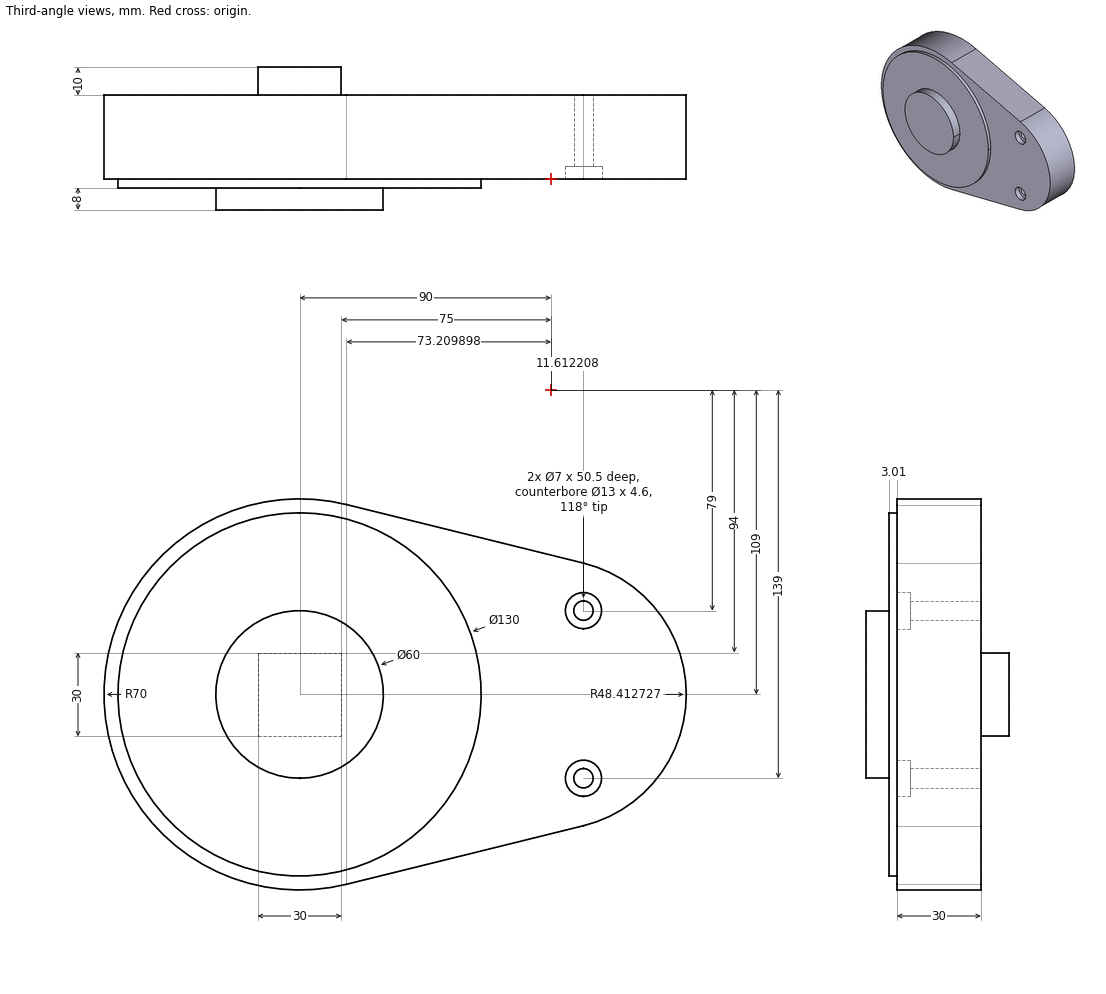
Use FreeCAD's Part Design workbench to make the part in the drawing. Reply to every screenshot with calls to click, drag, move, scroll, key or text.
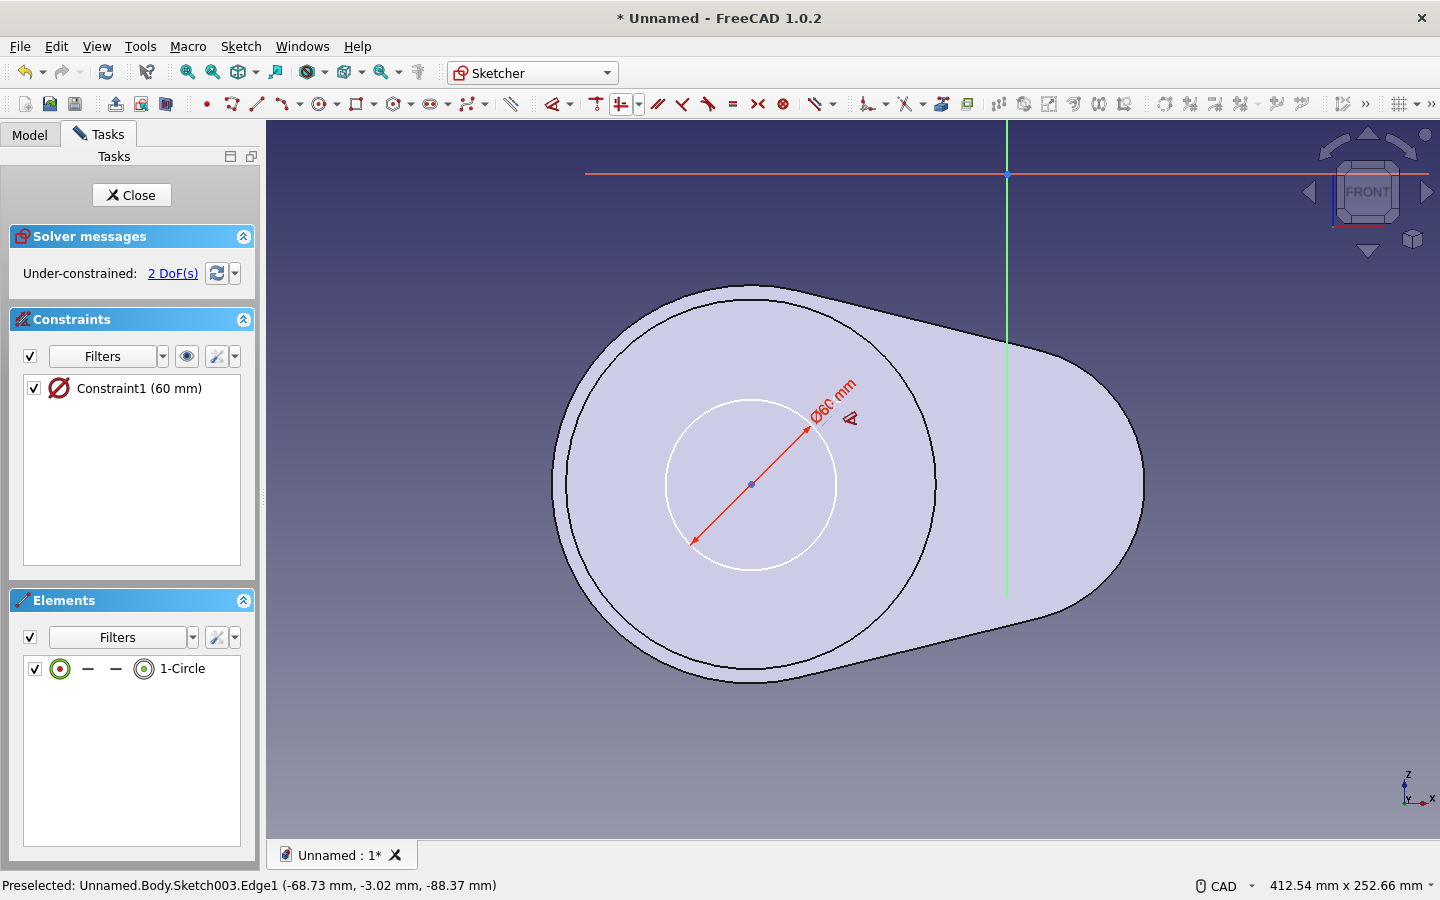
click(751, 485)
click(879, 519)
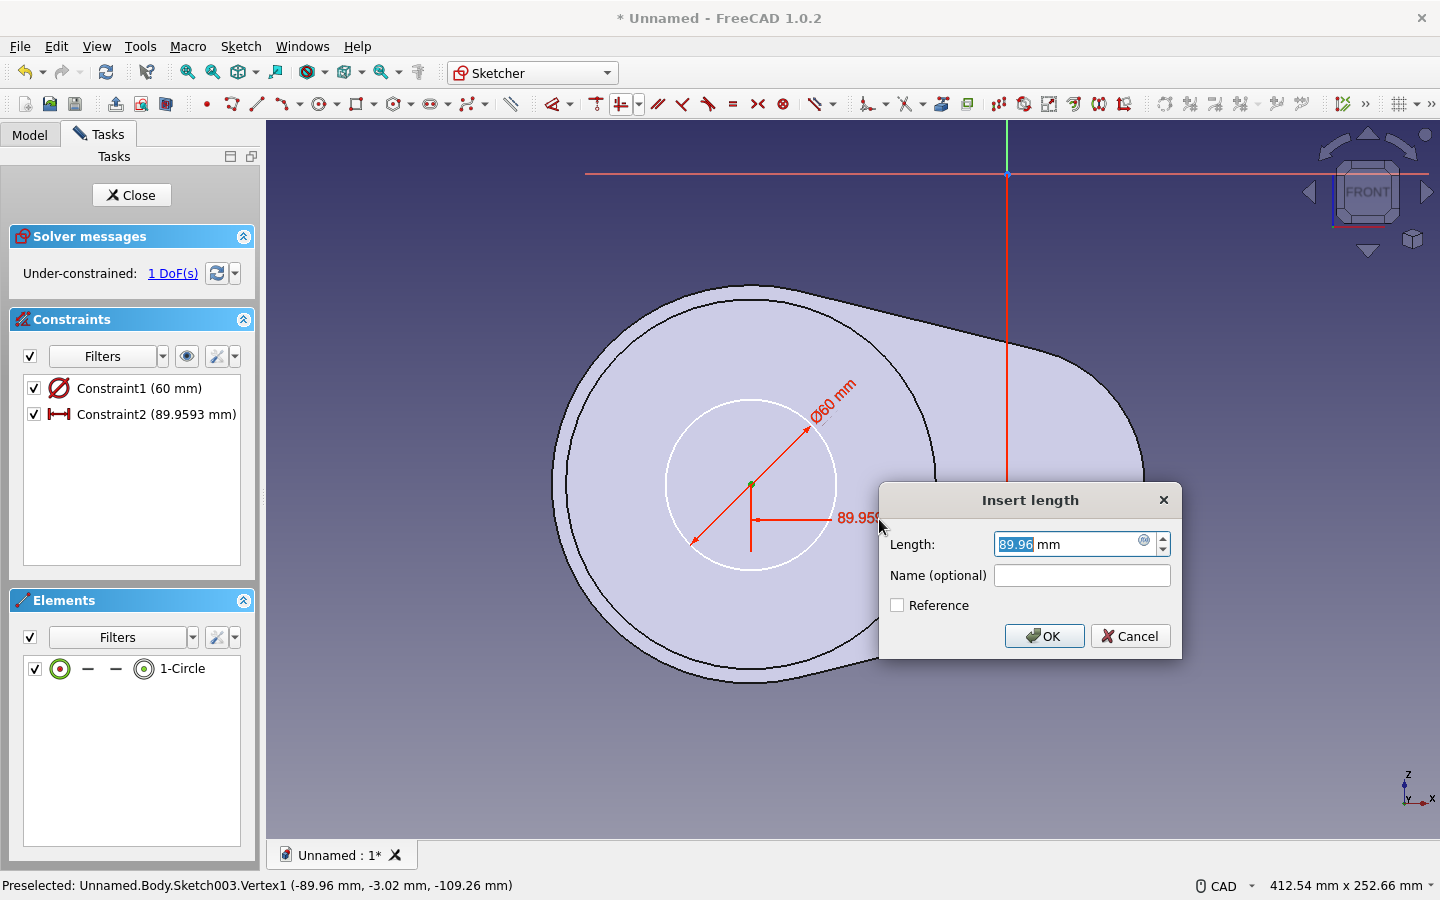
text(90)
key(Return)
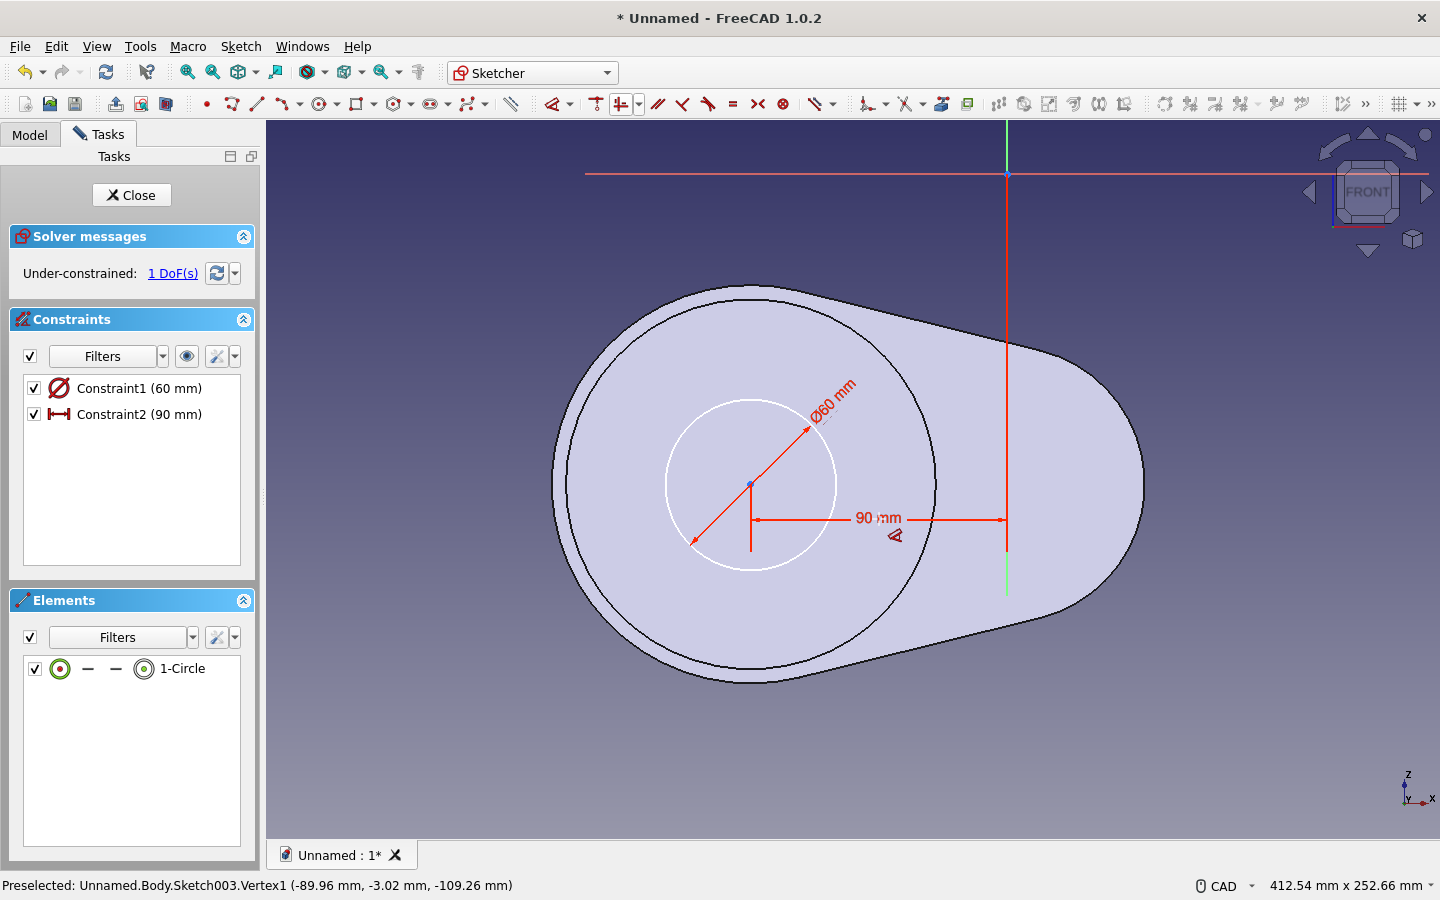
click(751, 485)
click(1041, 330)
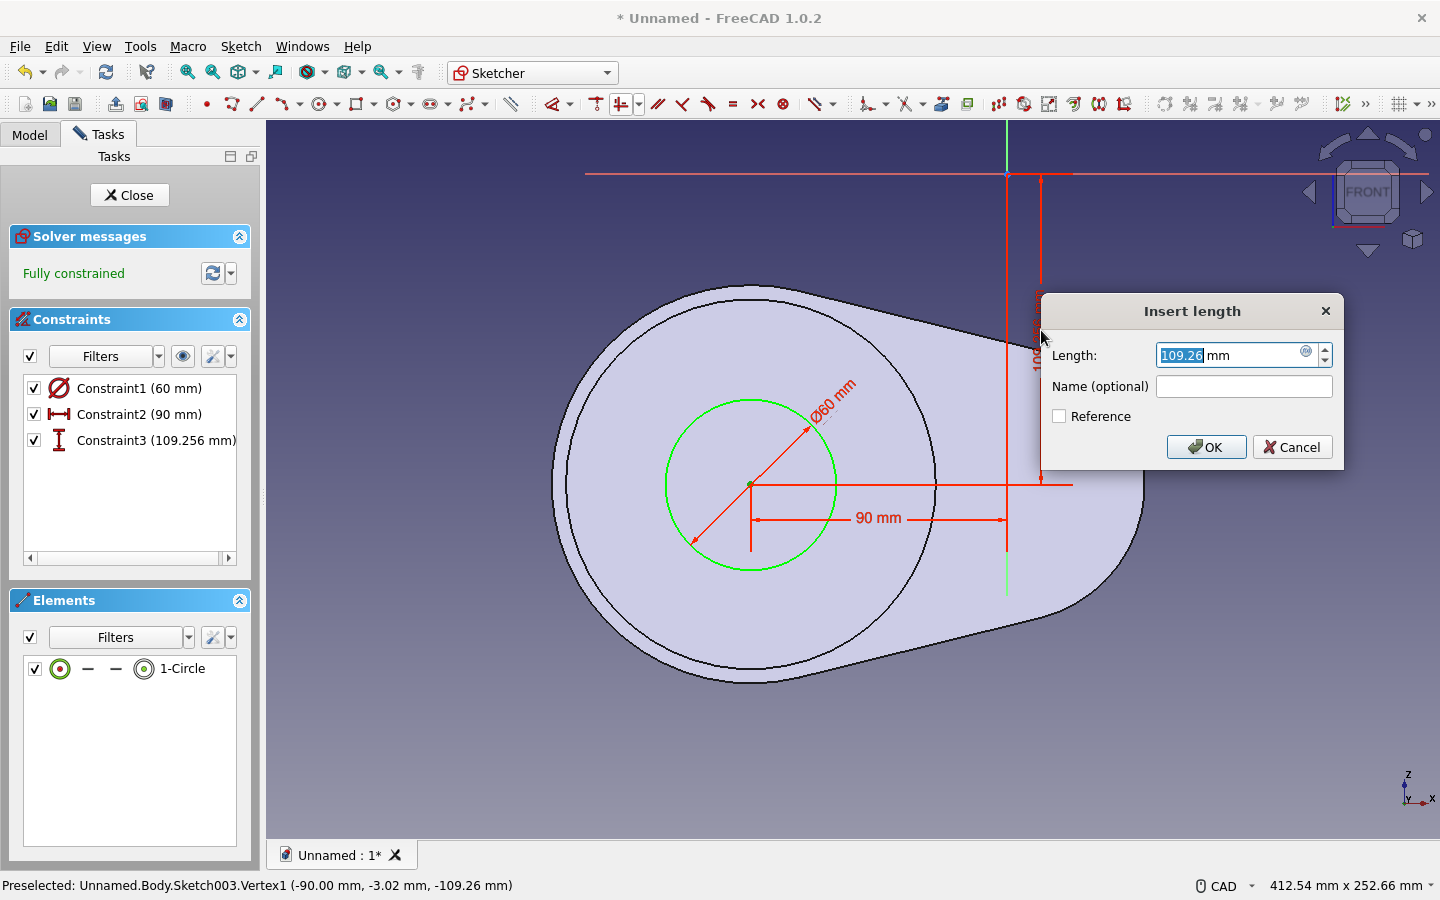
text(109)
key(Return)
key(Escape)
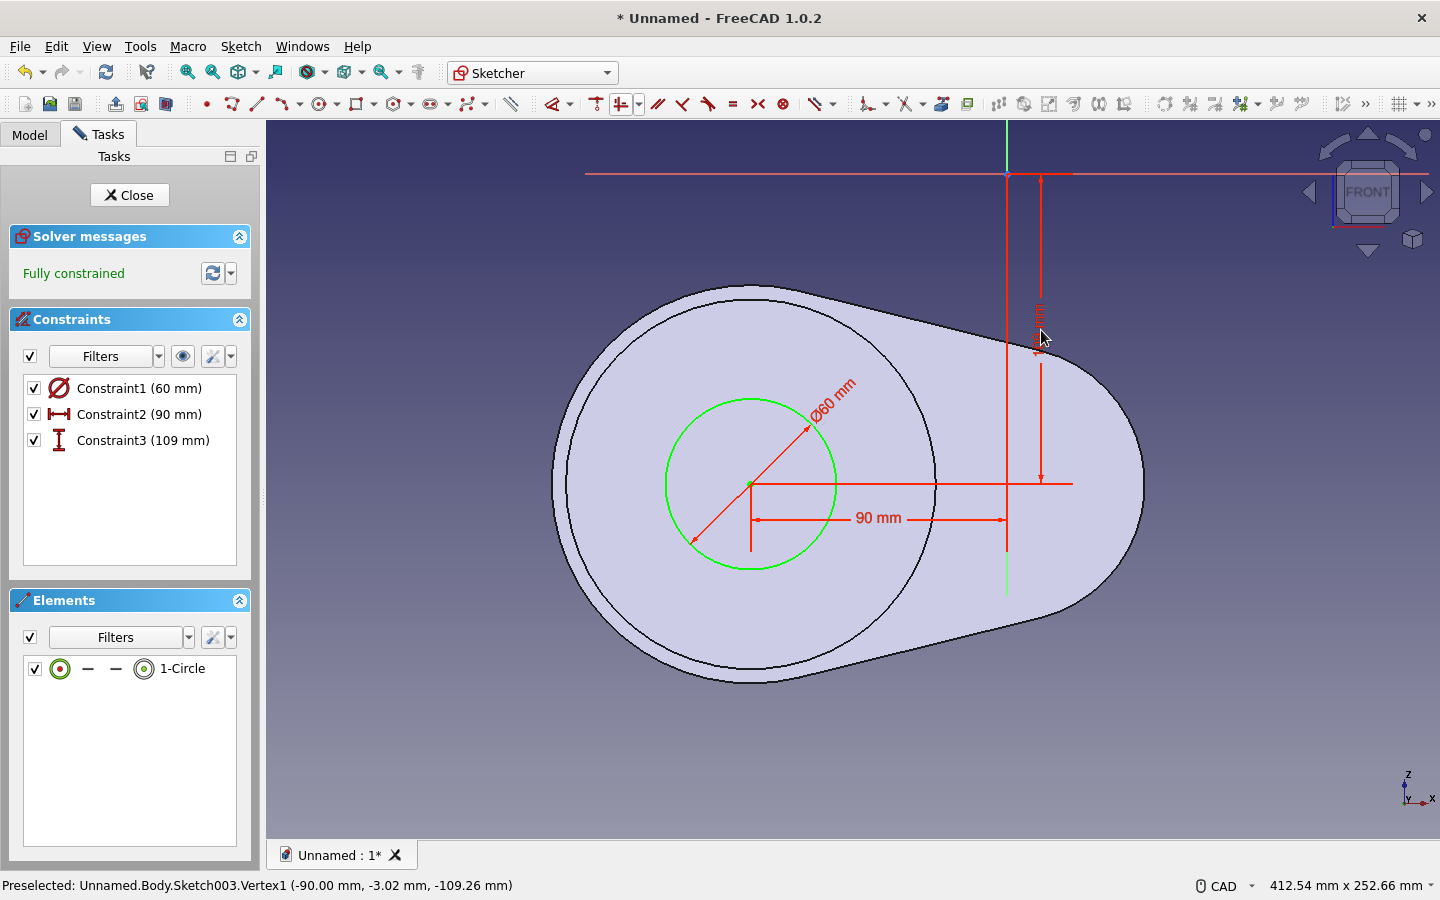
click(130, 195)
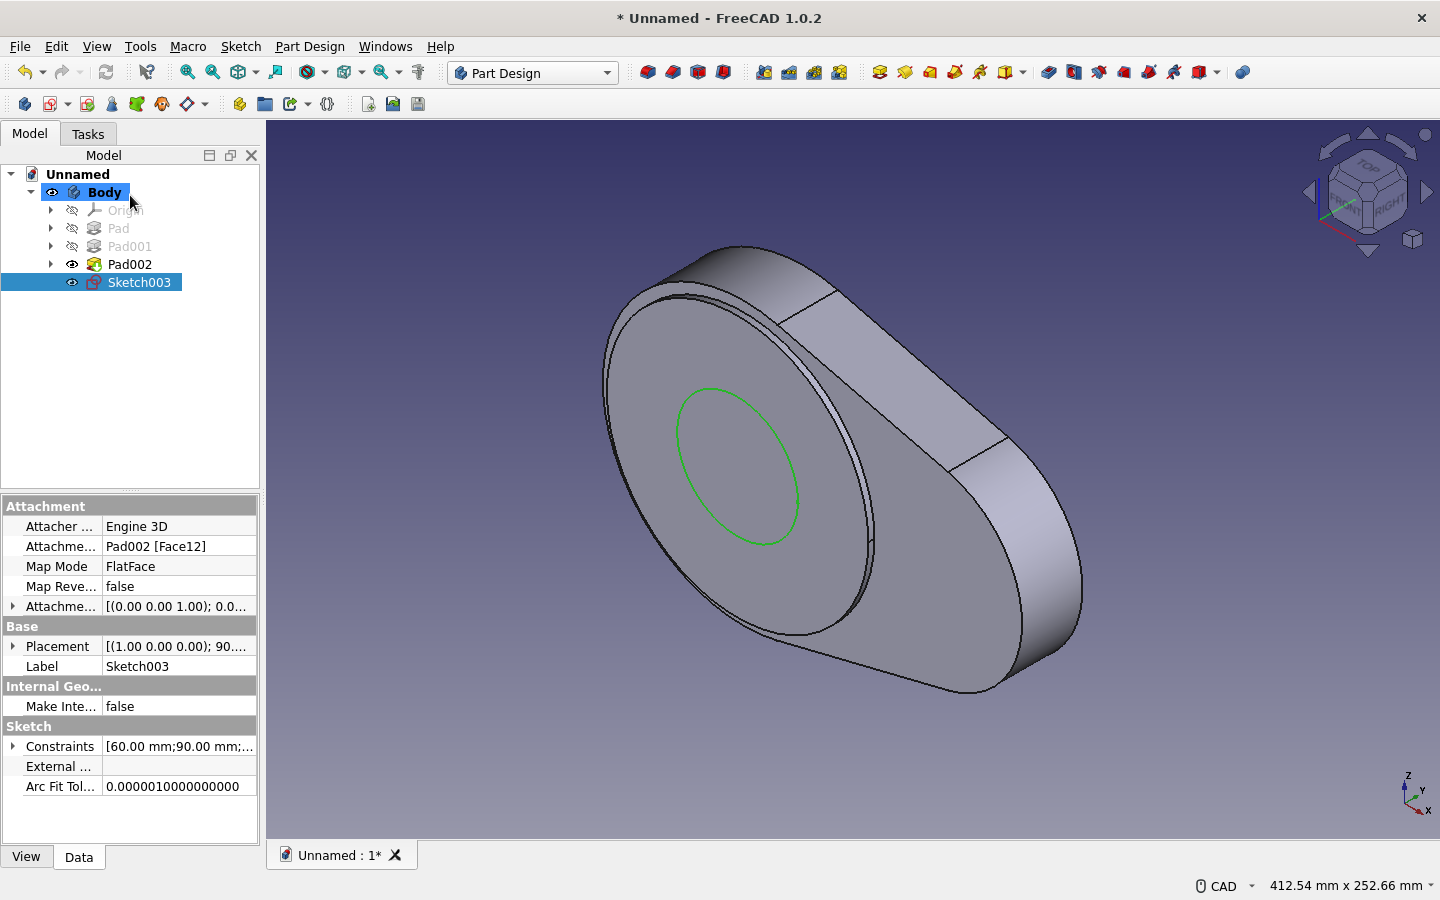
click(880, 72)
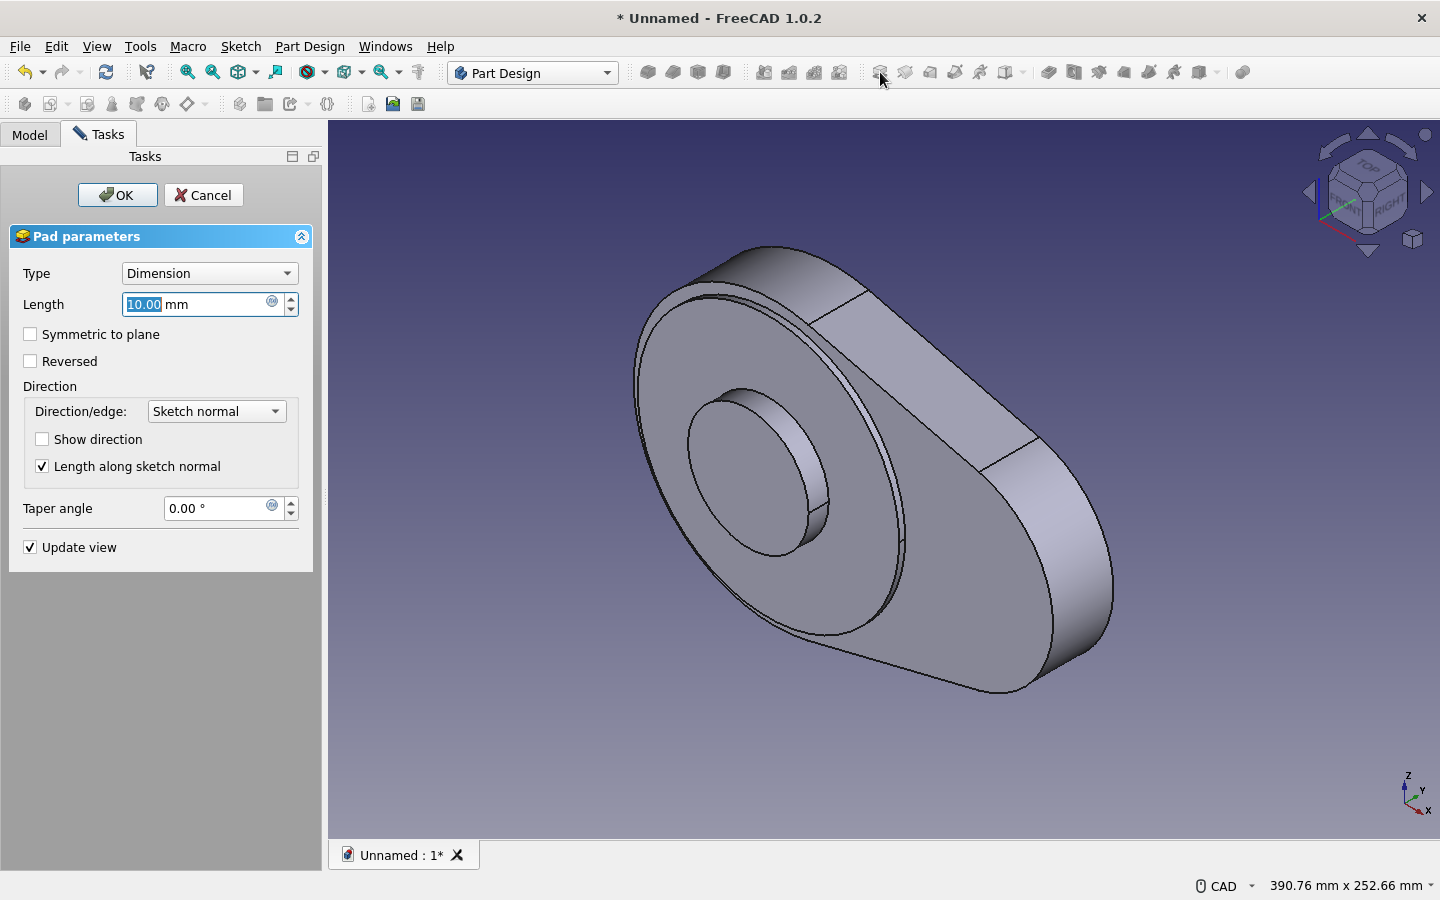
text(8)
key(Tab)